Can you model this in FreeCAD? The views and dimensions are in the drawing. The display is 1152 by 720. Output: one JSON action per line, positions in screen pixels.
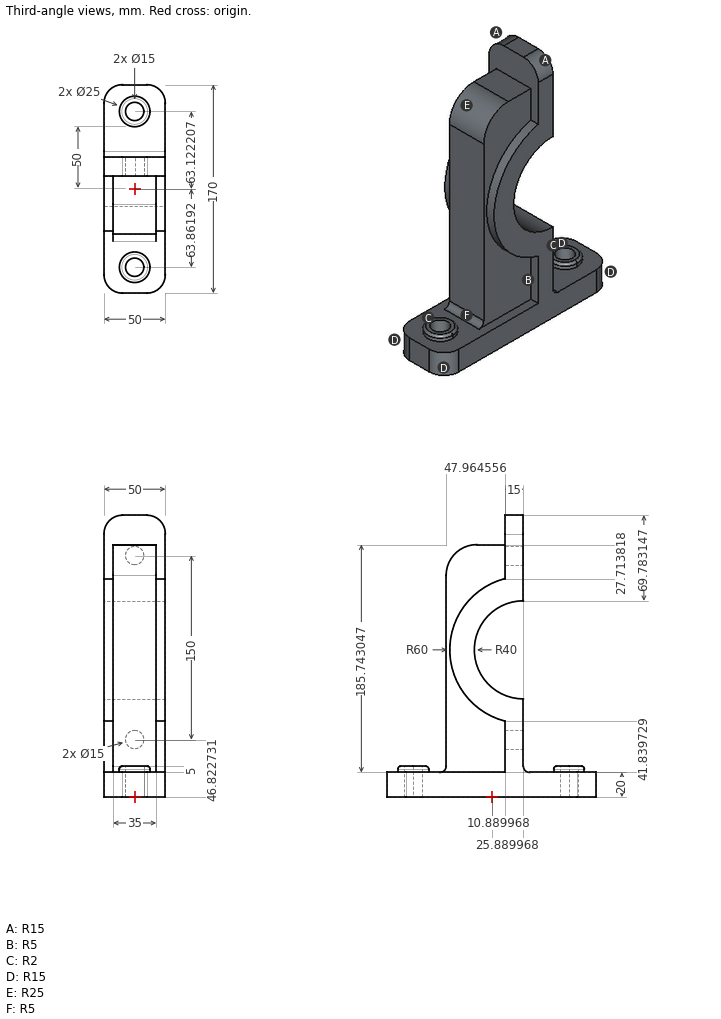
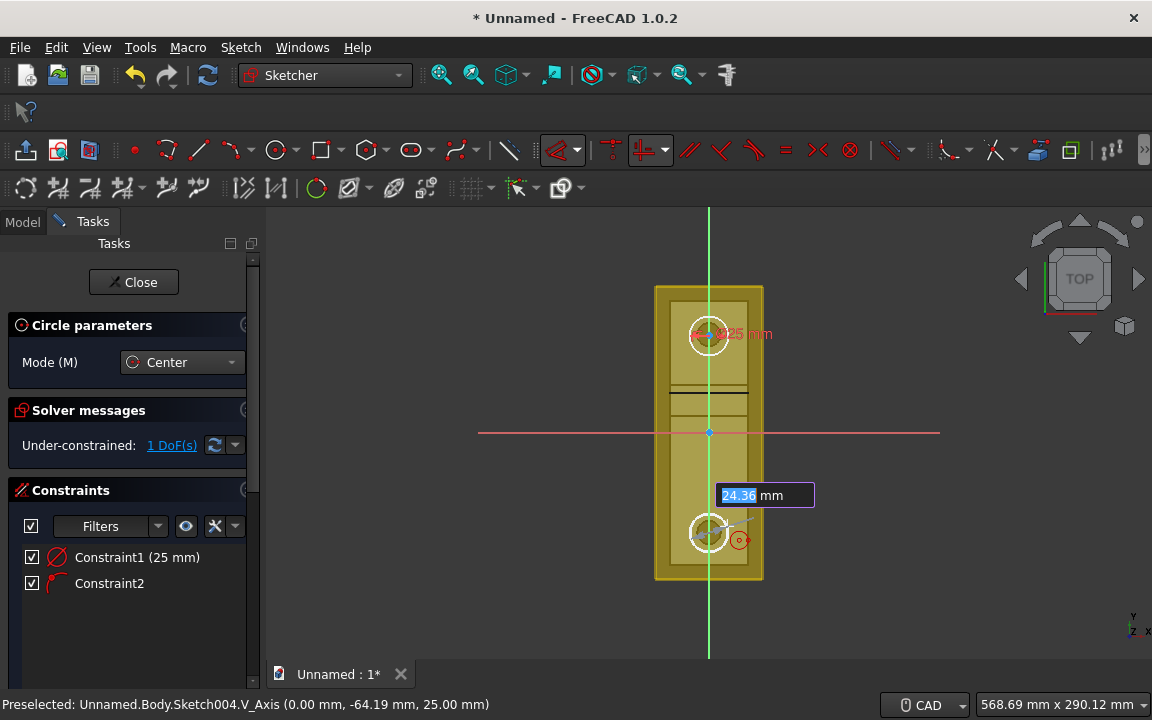
{"action": "type", "text": "25"}
{"action": "key", "text": "Return"}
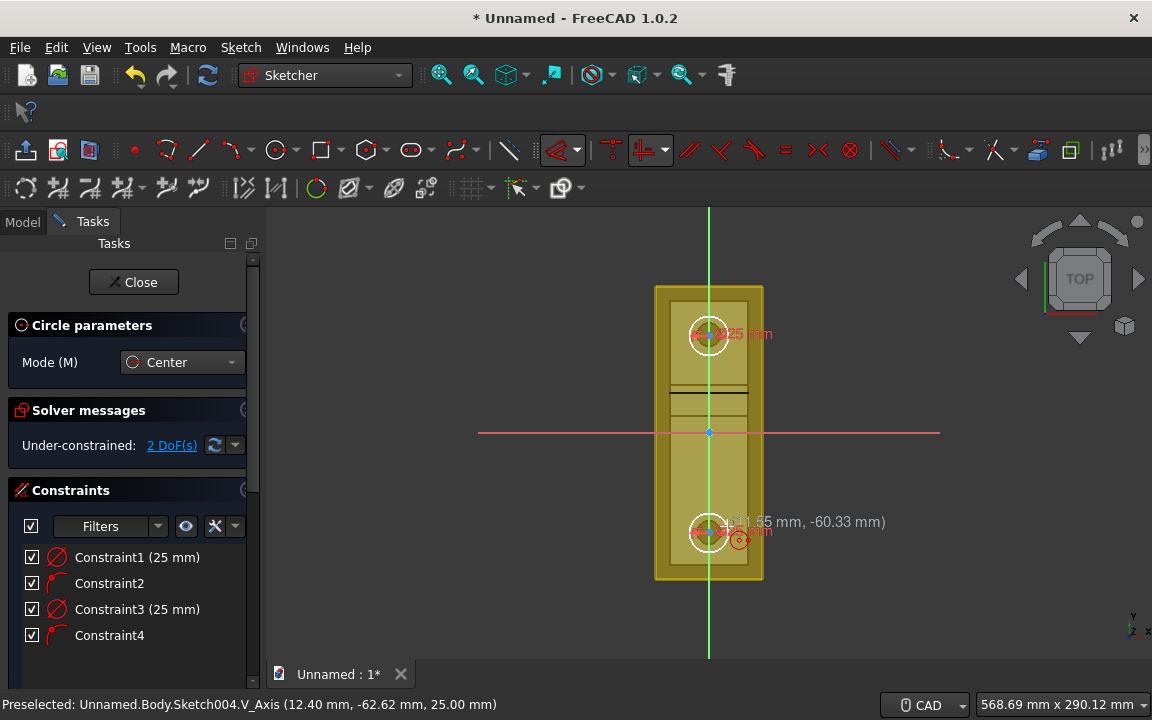
{"action": "scroll", "coordinate": [709, 335], "scroll_direction": "up", "scroll_amount": 4}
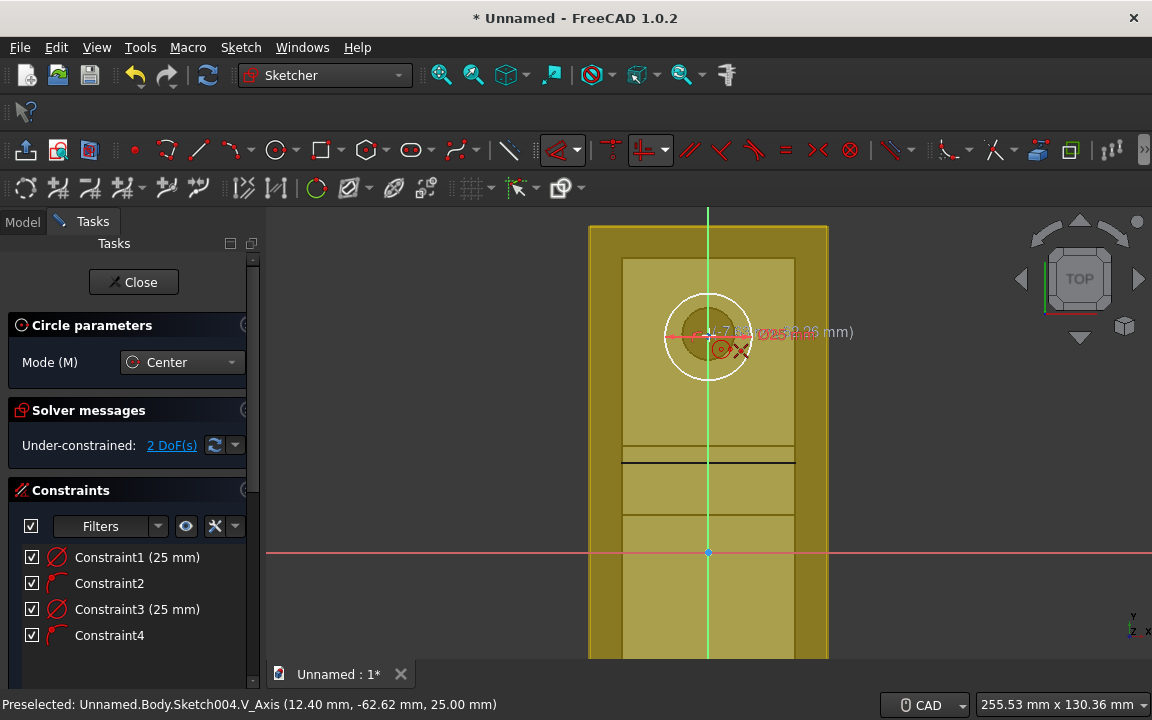
{"action": "left_click", "coordinate": [708, 337]}
{"action": "mouse_move", "coordinate": [727, 316]}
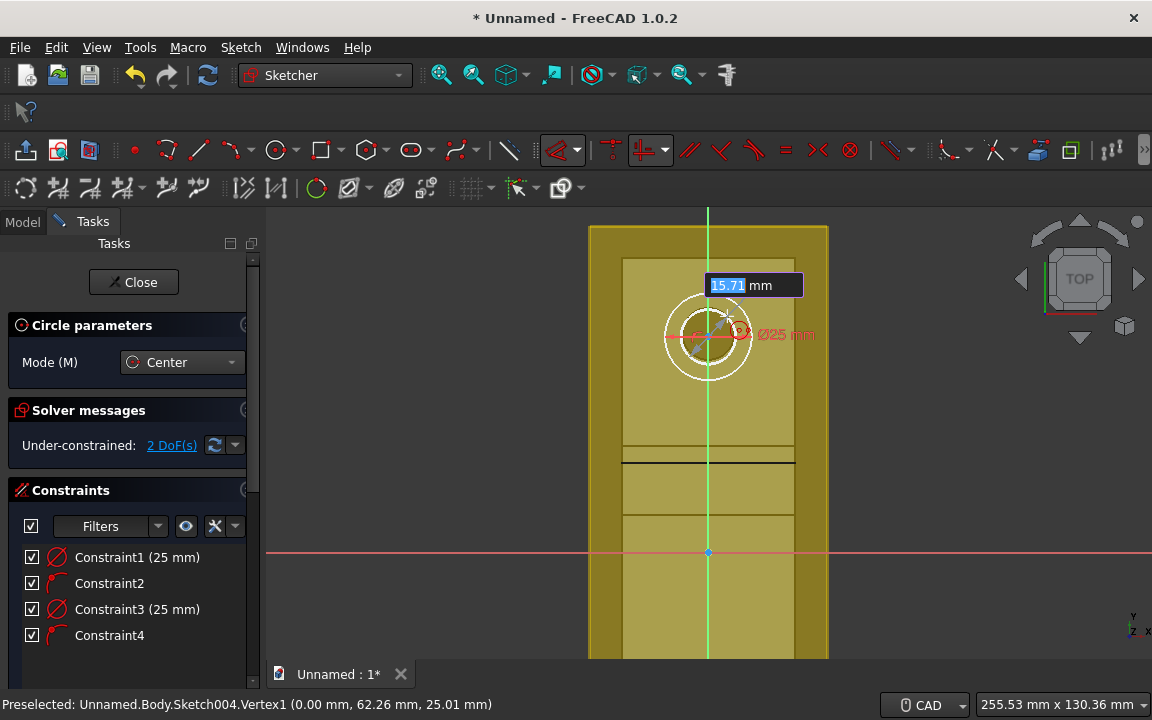
{"action": "type", "text": "15"}
{"action": "key", "text": "Return"}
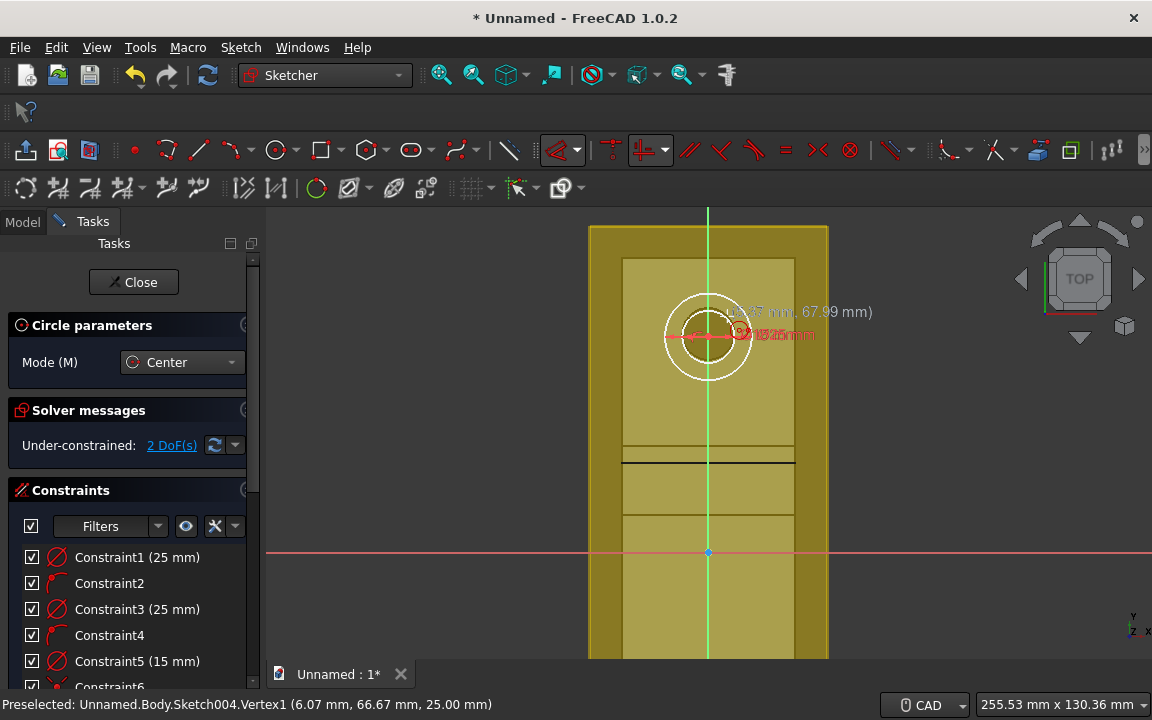
{"action": "scroll", "coordinate": [558, 286], "scroll_direction": "down", "scroll_amount": 3}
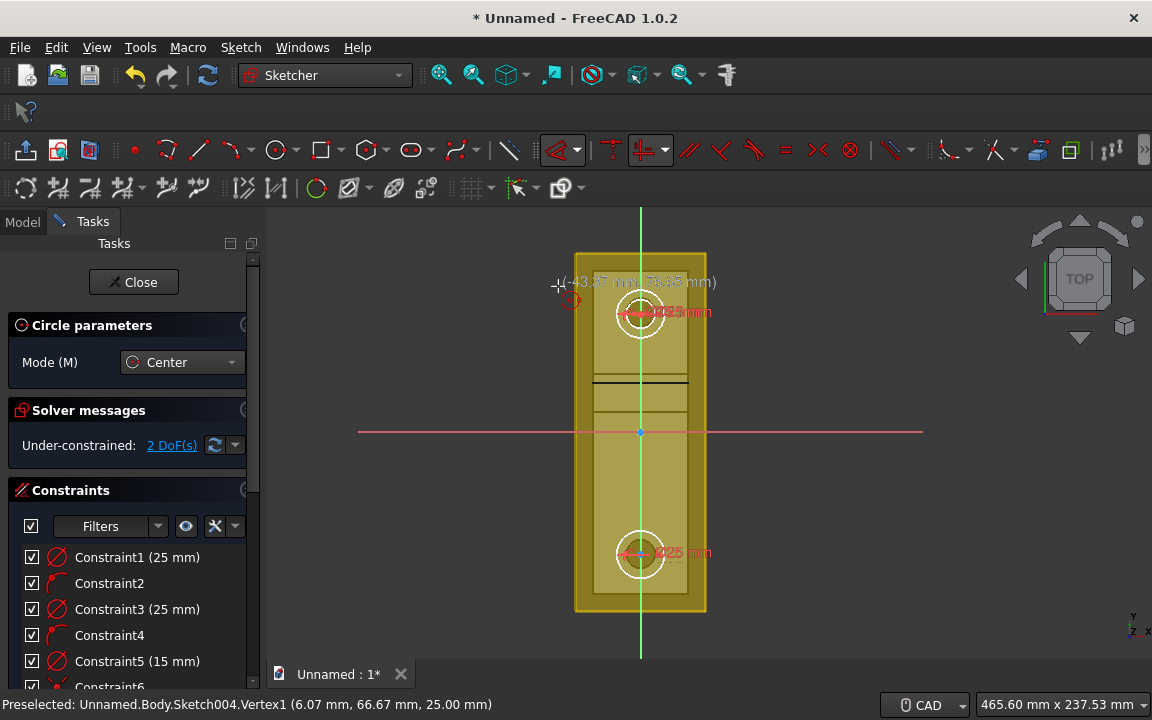
{"action": "scroll", "coordinate": [641, 554], "scroll_direction": "up", "scroll_amount": 3}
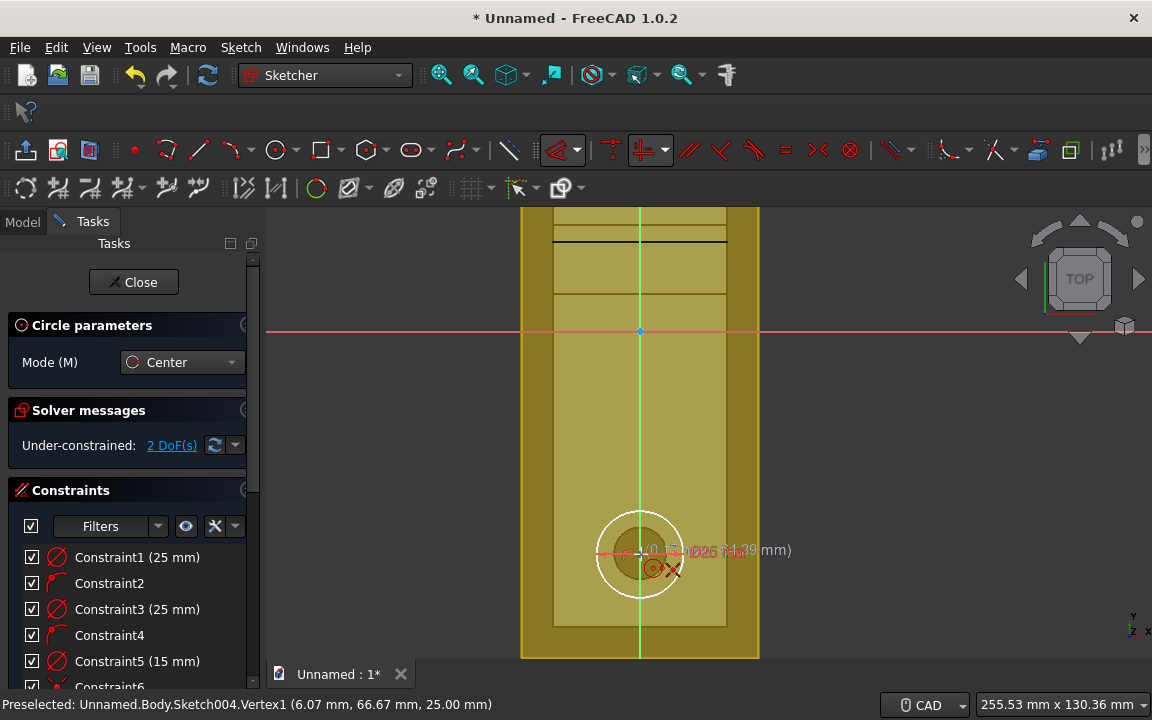
{"action": "left_click", "coordinate": [640, 554]}
{"action": "mouse_move", "coordinate": [658, 535]}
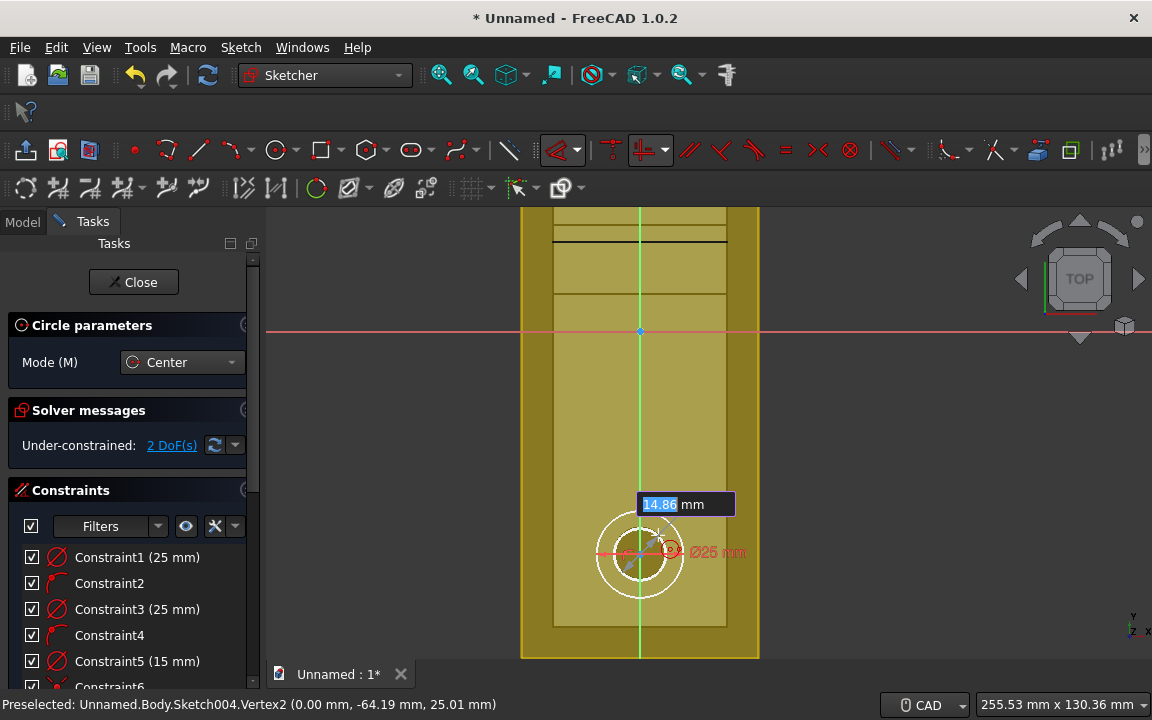
{"action": "type", "text": "15"}
{"action": "key", "text": "Return"}
{"action": "key", "text": "Escape"}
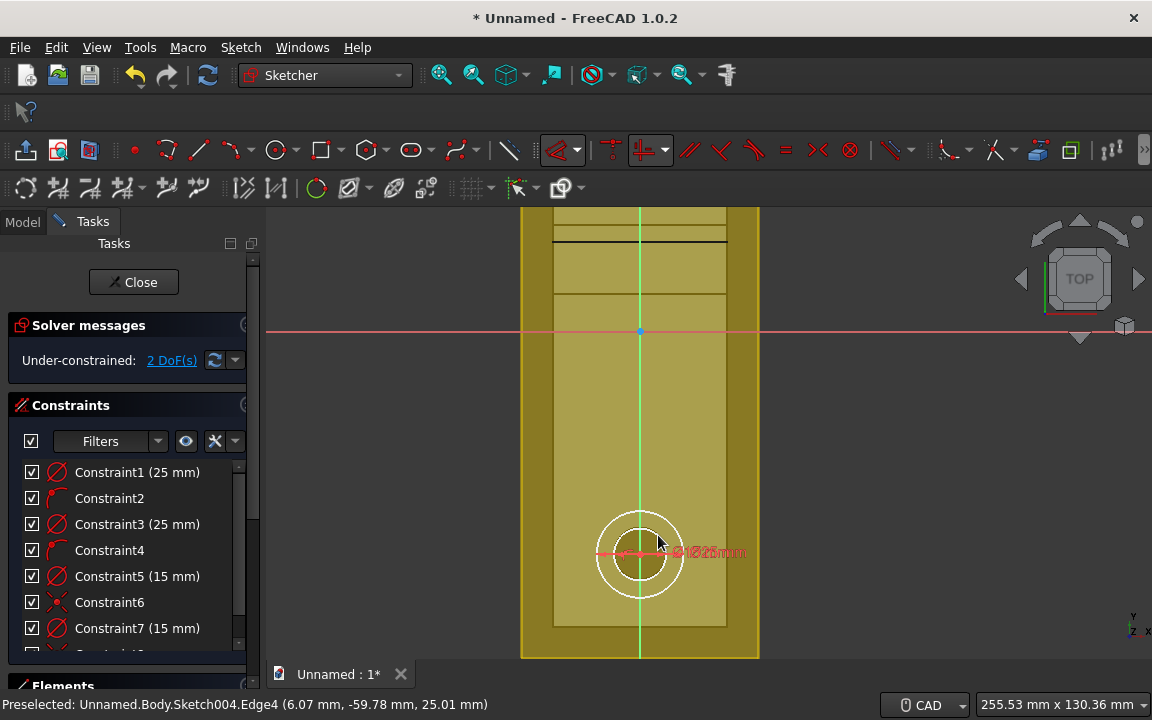
{"action": "left_click", "coordinate": [640, 554]}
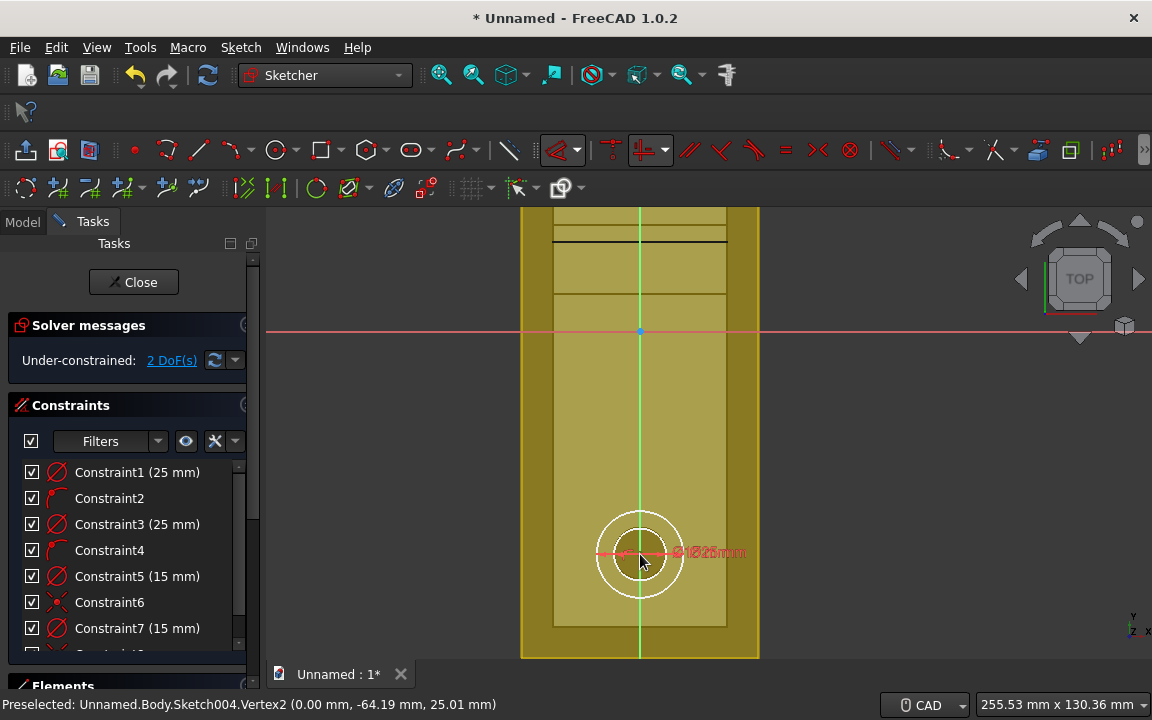
{"action": "key", "text": "i"}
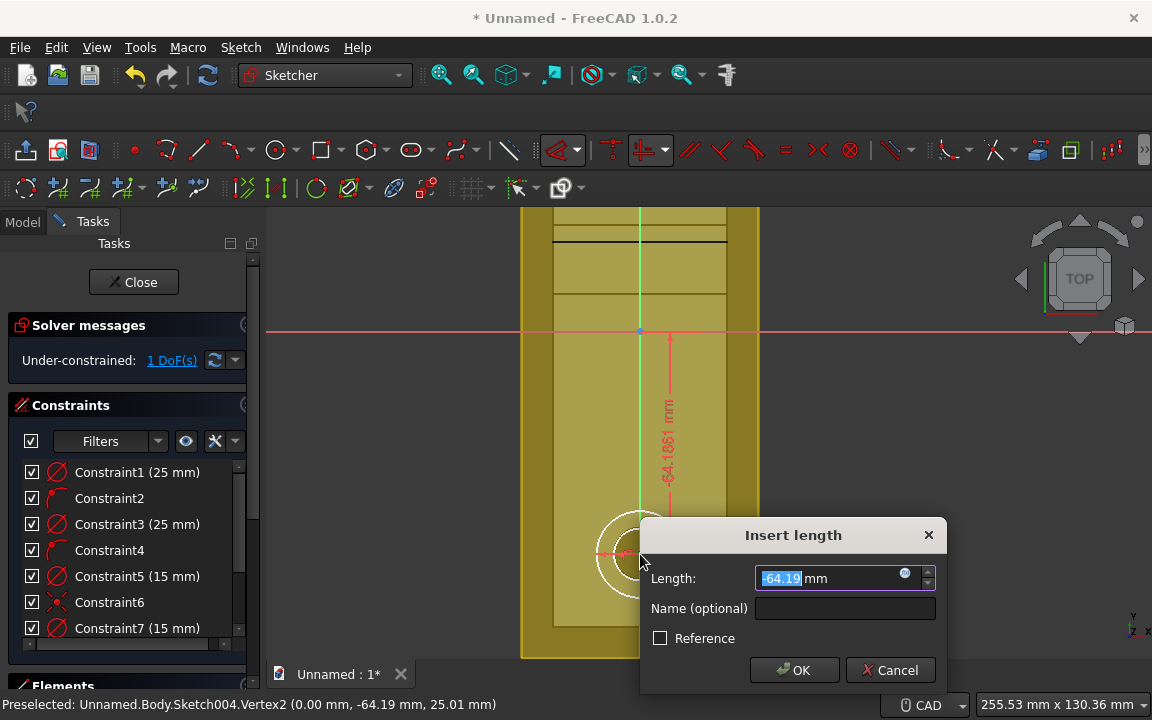
{"action": "type", "text": "-63.86192"}
{"action": "key", "text": "Return"}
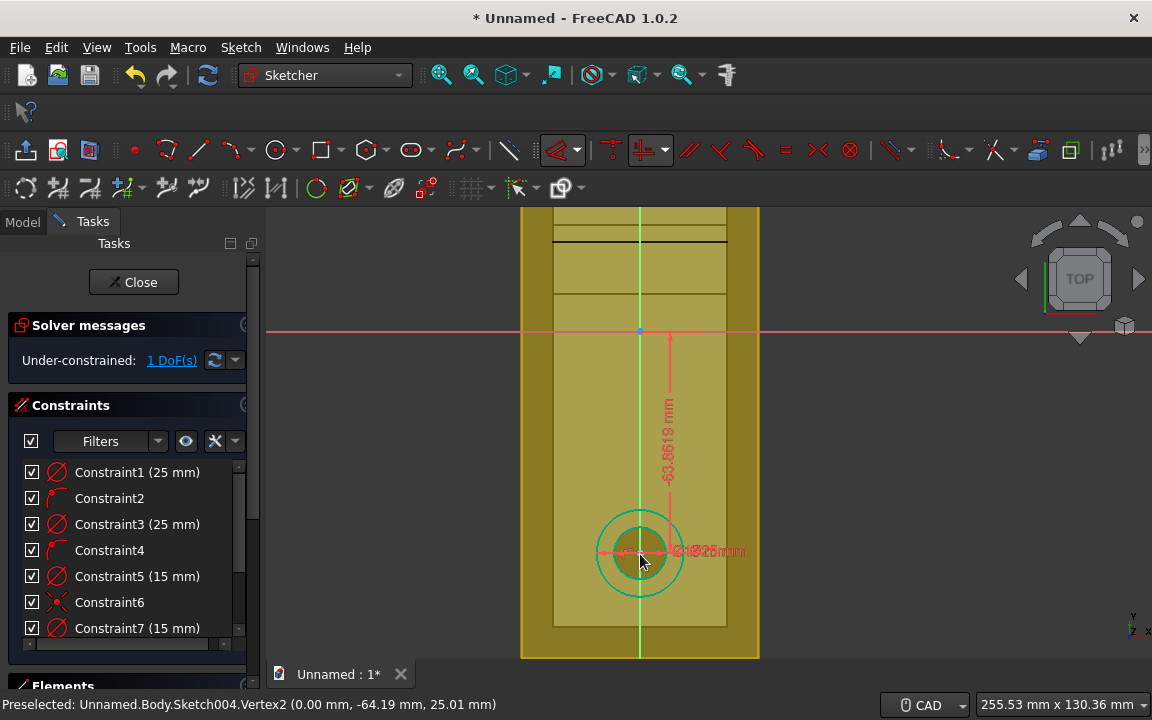
{"action": "scroll", "coordinate": [641, 554], "scroll_direction": "down", "scroll_amount": 3}